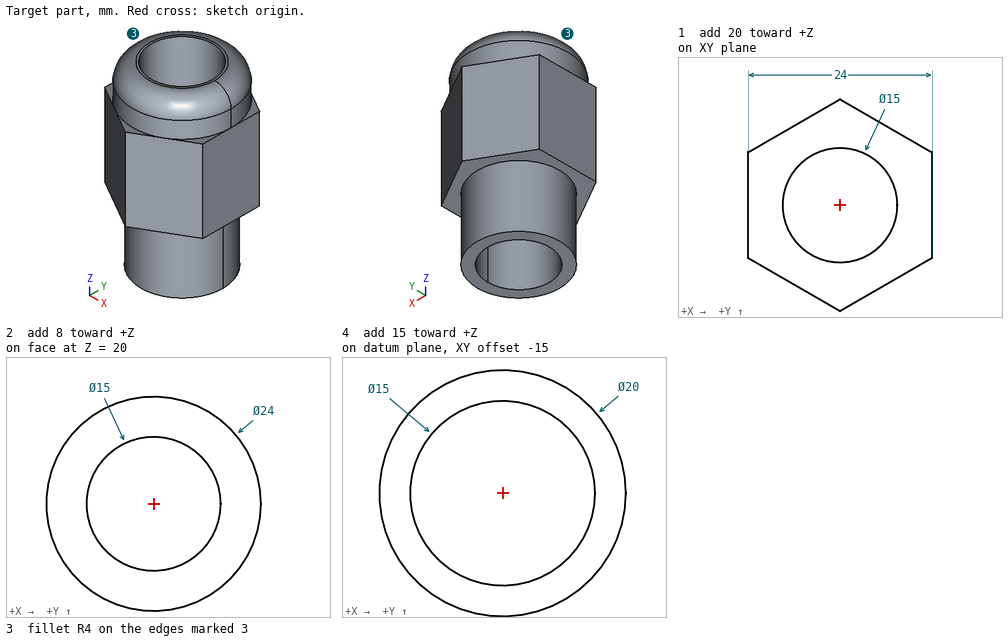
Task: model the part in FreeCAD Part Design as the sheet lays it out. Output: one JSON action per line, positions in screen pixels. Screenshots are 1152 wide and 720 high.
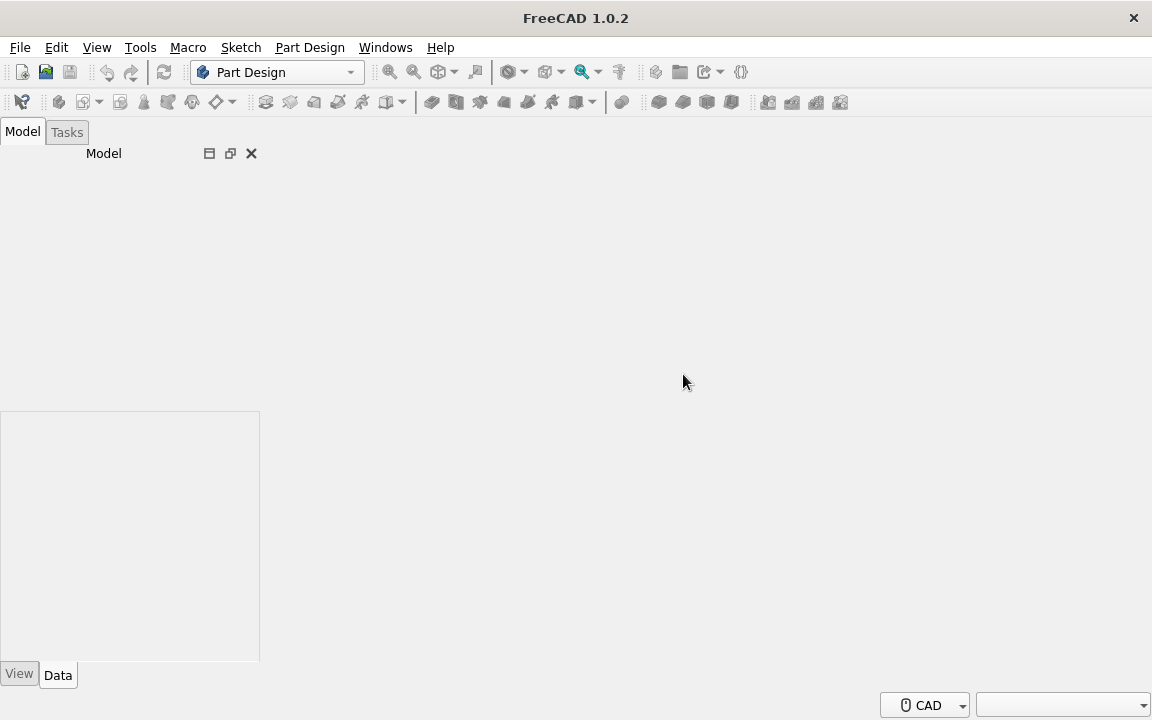
{"action": "left_click", "coordinate": [22, 72]}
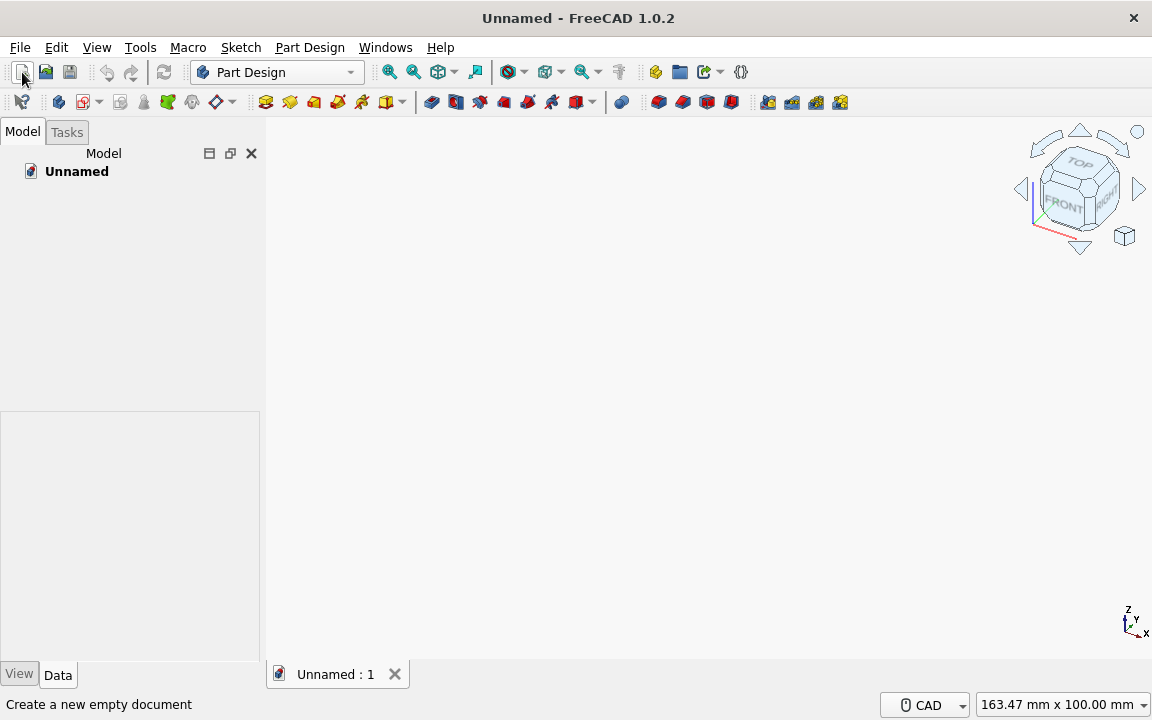
{"action": "left_click", "coordinate": [84, 102]}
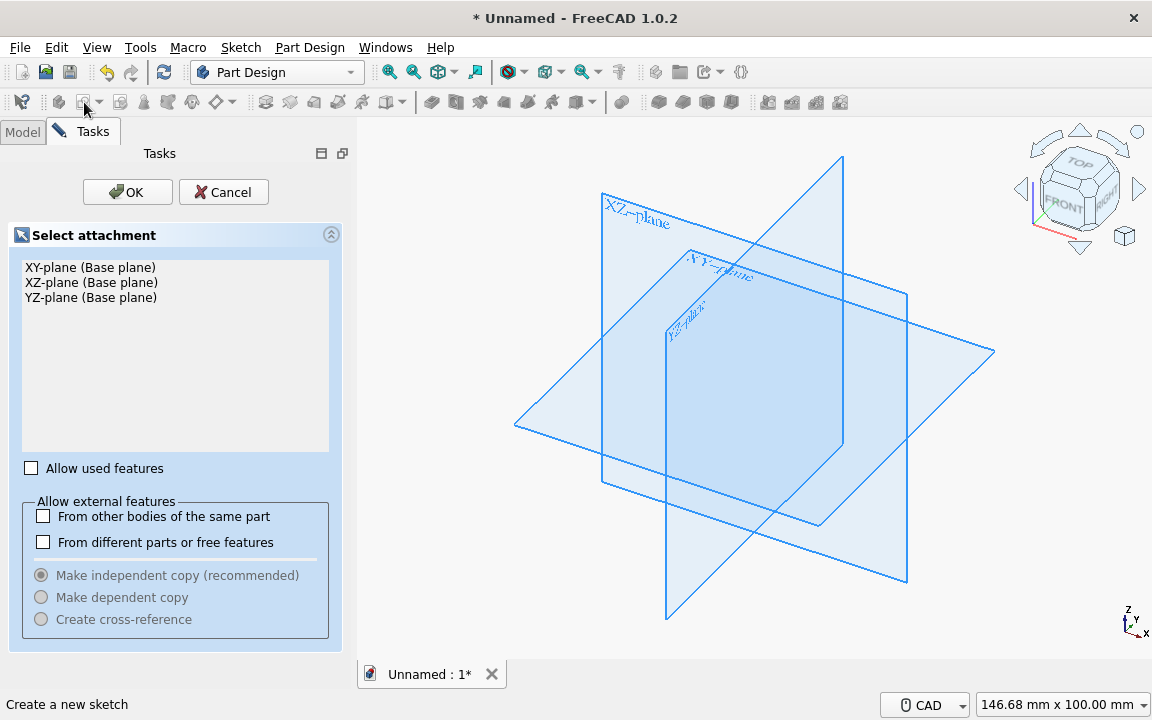
{"action": "left_click", "coordinate": [82, 268]}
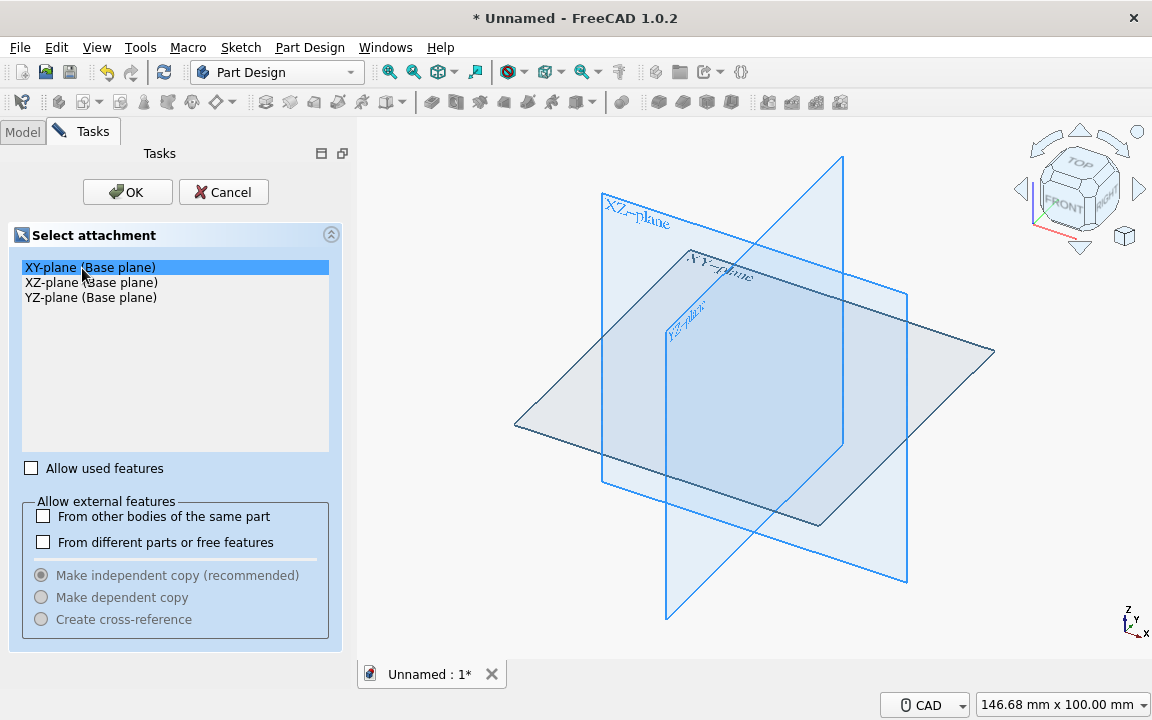
{"action": "left_click", "coordinate": [128, 192]}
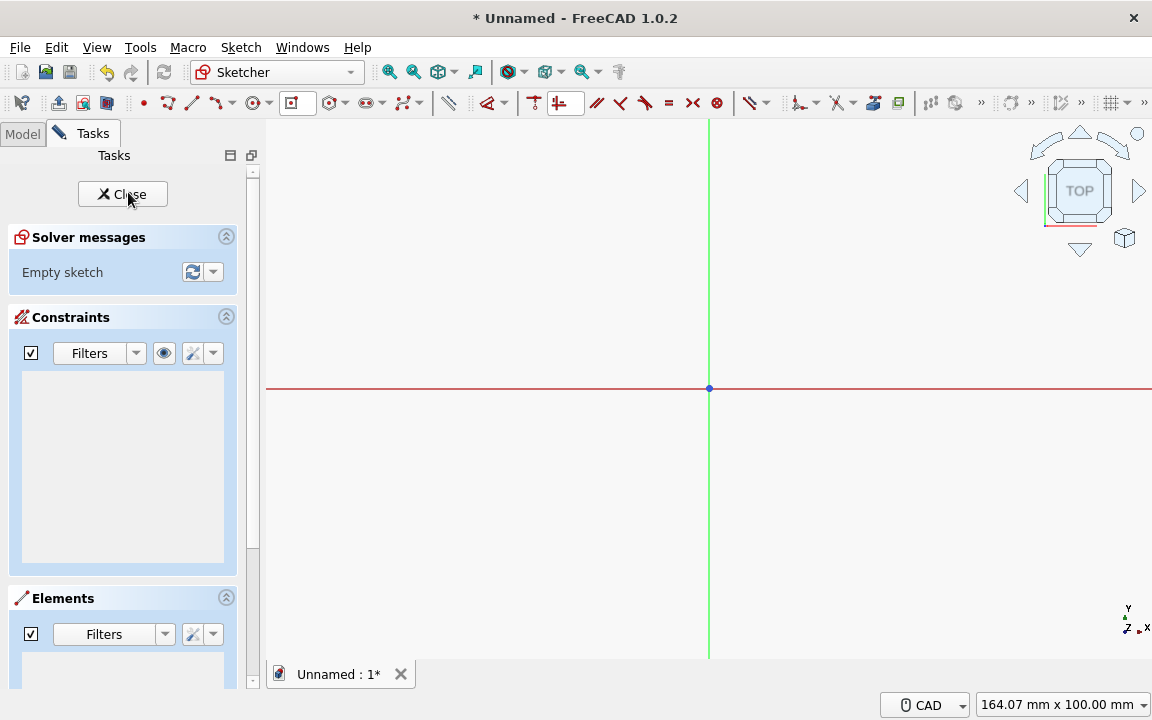
{"action": "scroll", "coordinate": [765, 389], "scroll_direction": "up", "scroll_amount": 4}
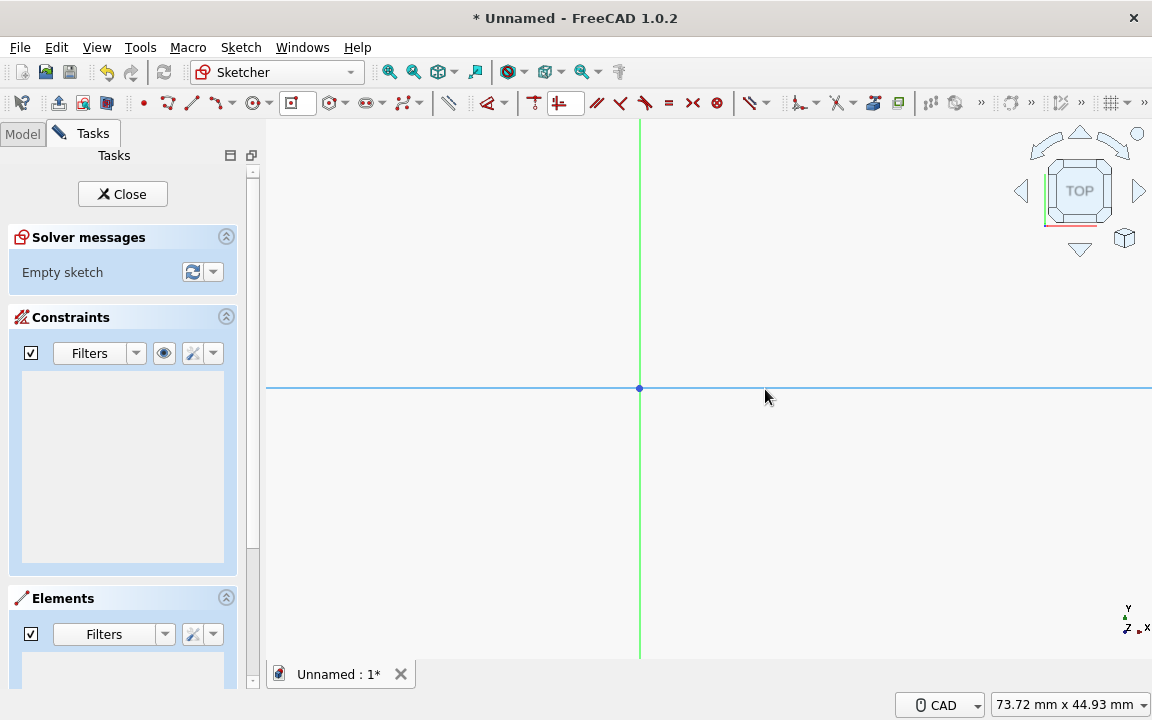
{"action": "key", "text": "g p 6"}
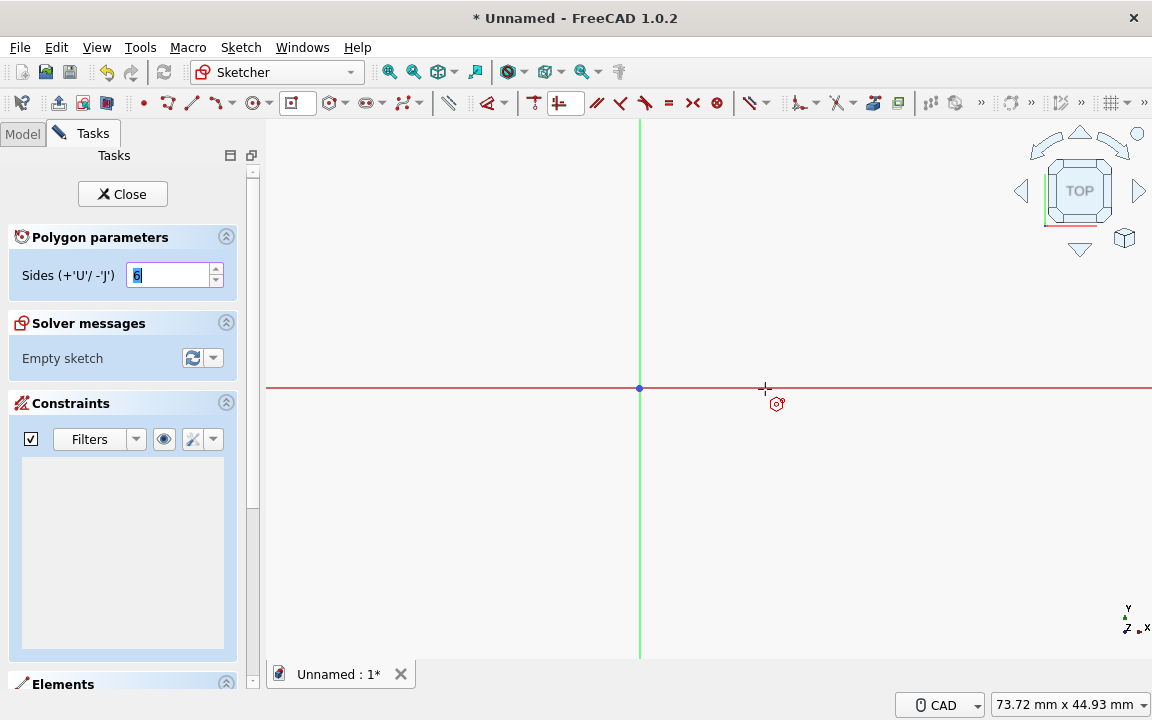
{"action": "left_click", "coordinate": [640, 388]}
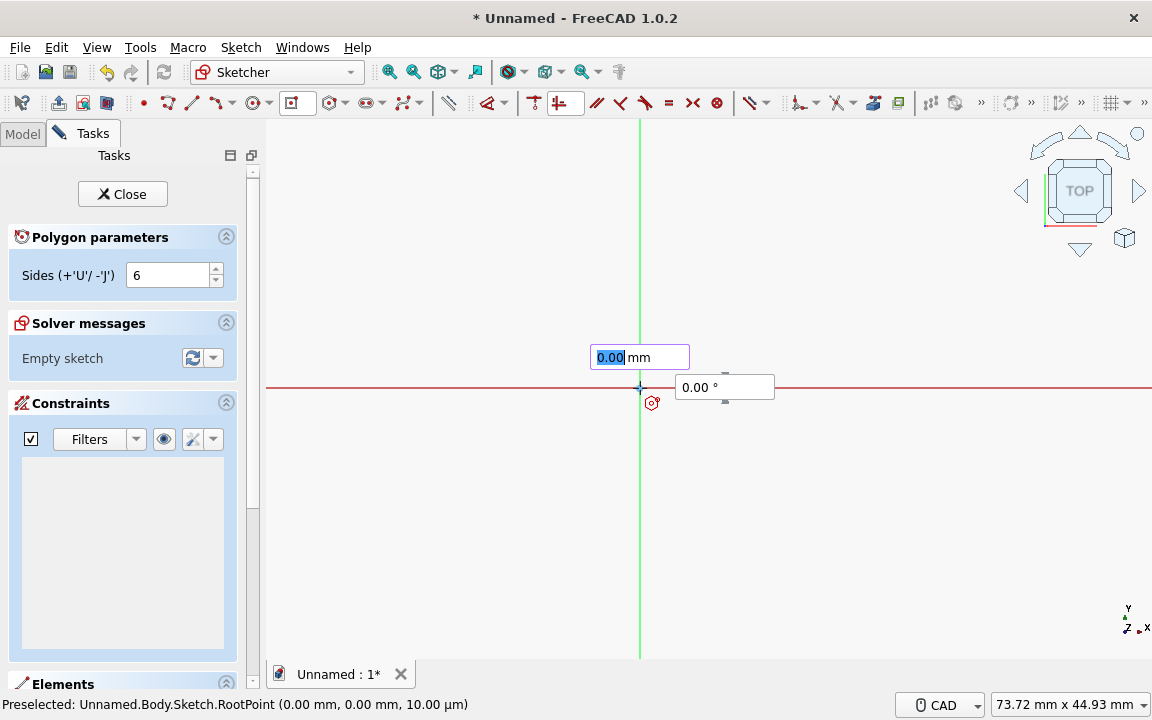
{"action": "left_click", "coordinate": [640, 222]}
{"action": "right_click", "coordinate": [640, 222]}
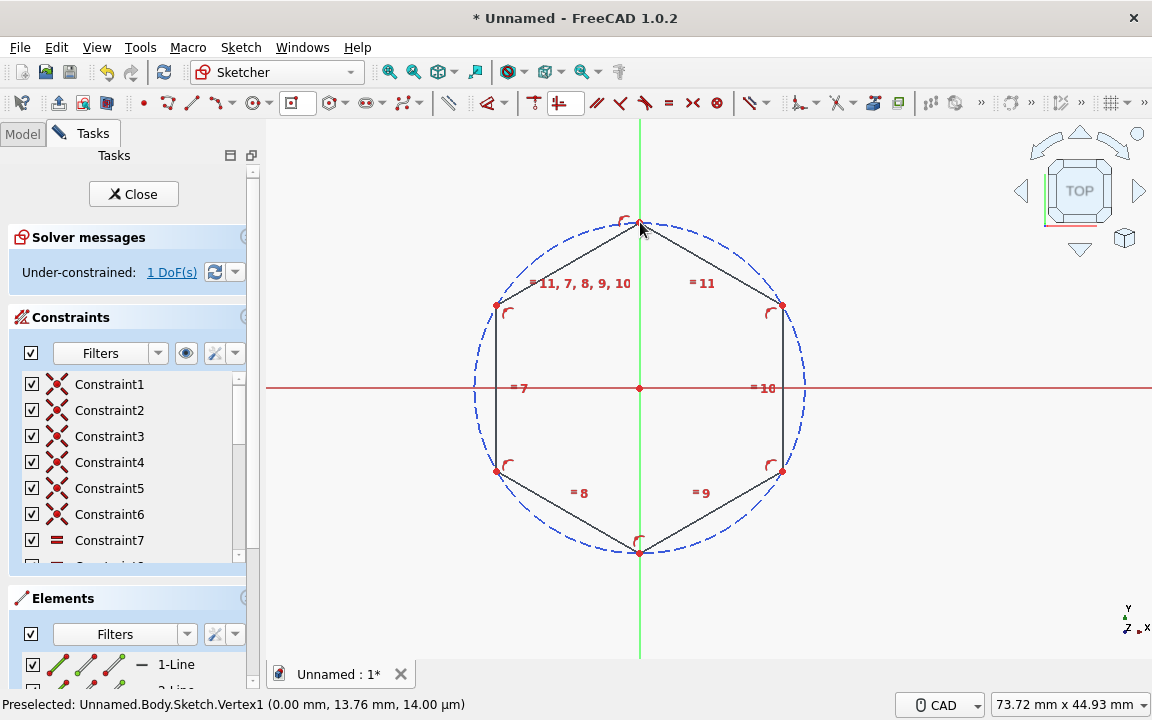
{"action": "left_click", "coordinate": [254, 104]}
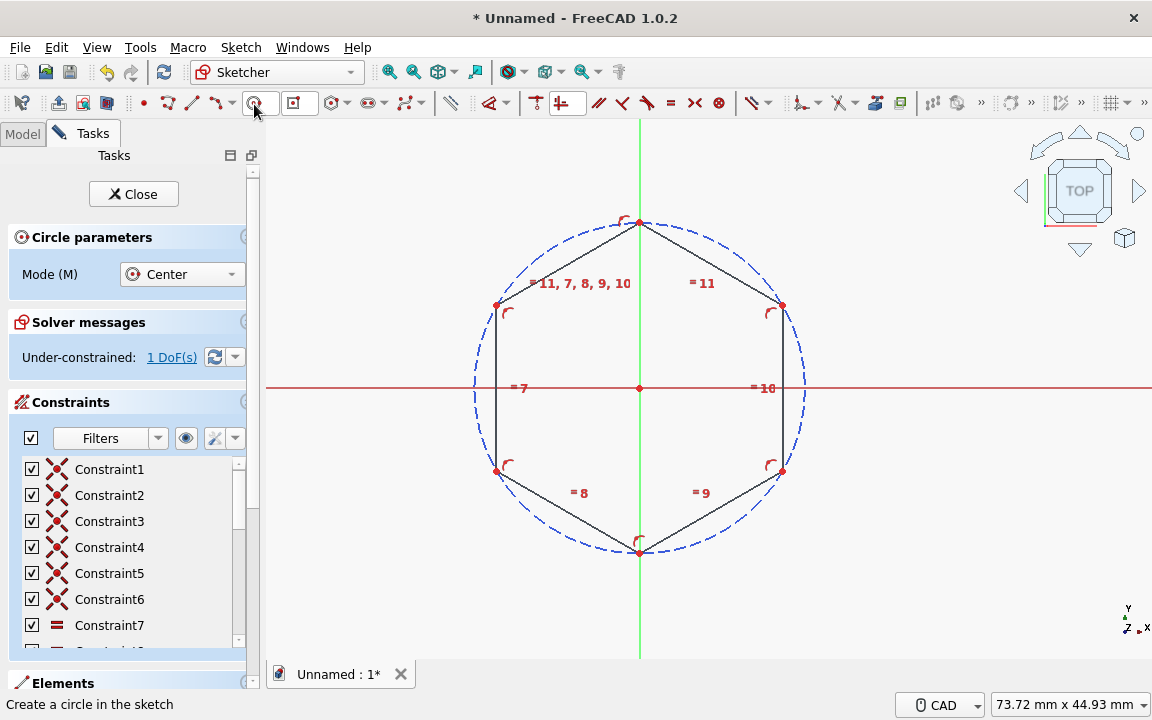
{"action": "left_click", "coordinate": [640, 388]}
{"action": "mouse_move", "coordinate": [703, 325]}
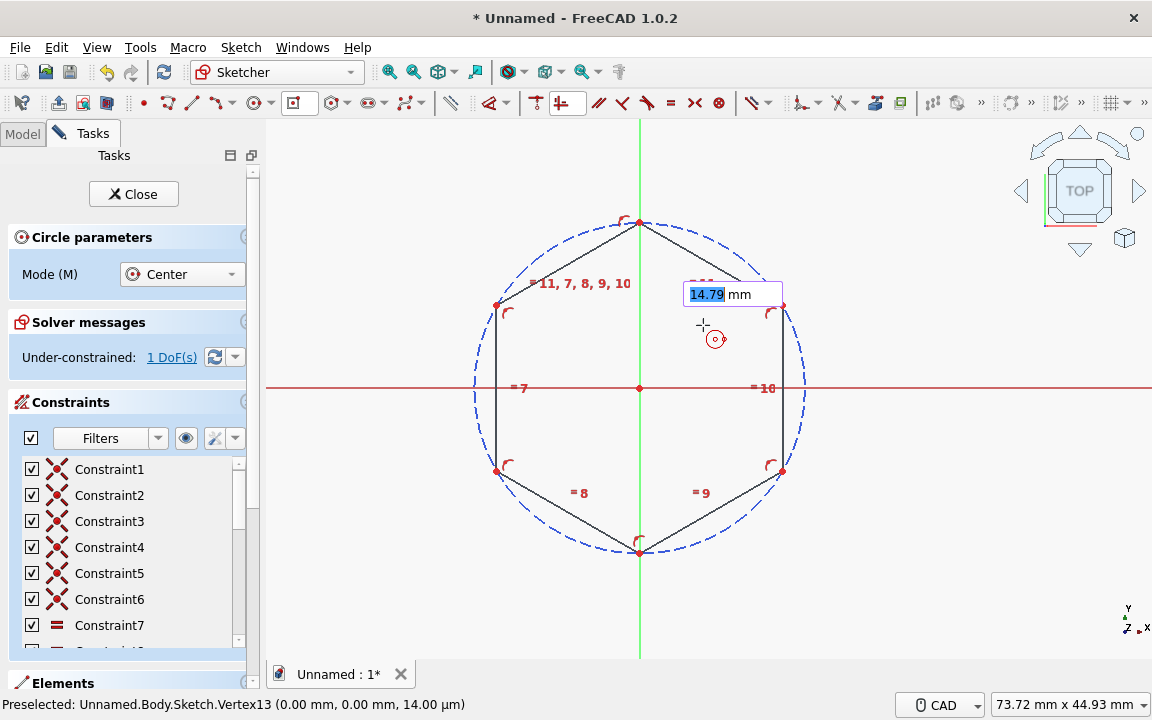
{"action": "type", "text": "15"}
{"action": "key", "text": "Return"}
{"action": "key", "text": "Escape"}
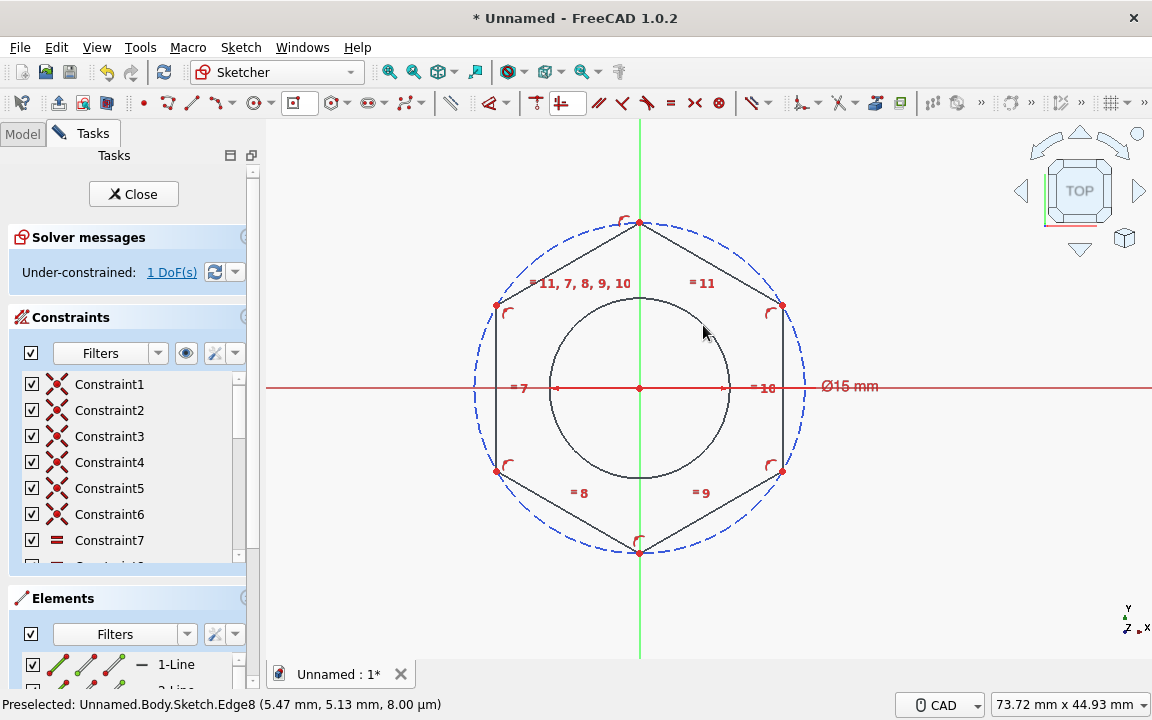
{"action": "left_click", "coordinate": [490, 104]}